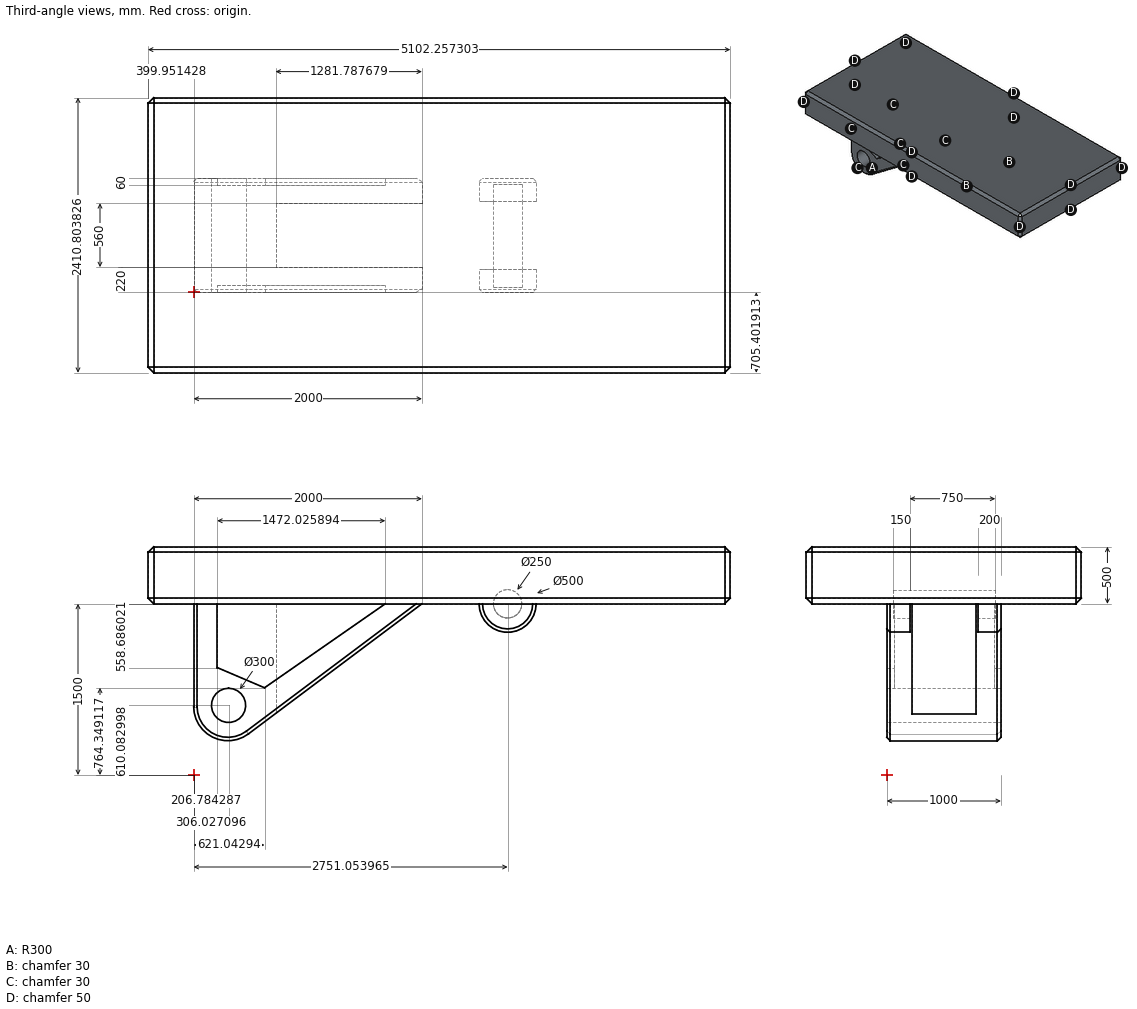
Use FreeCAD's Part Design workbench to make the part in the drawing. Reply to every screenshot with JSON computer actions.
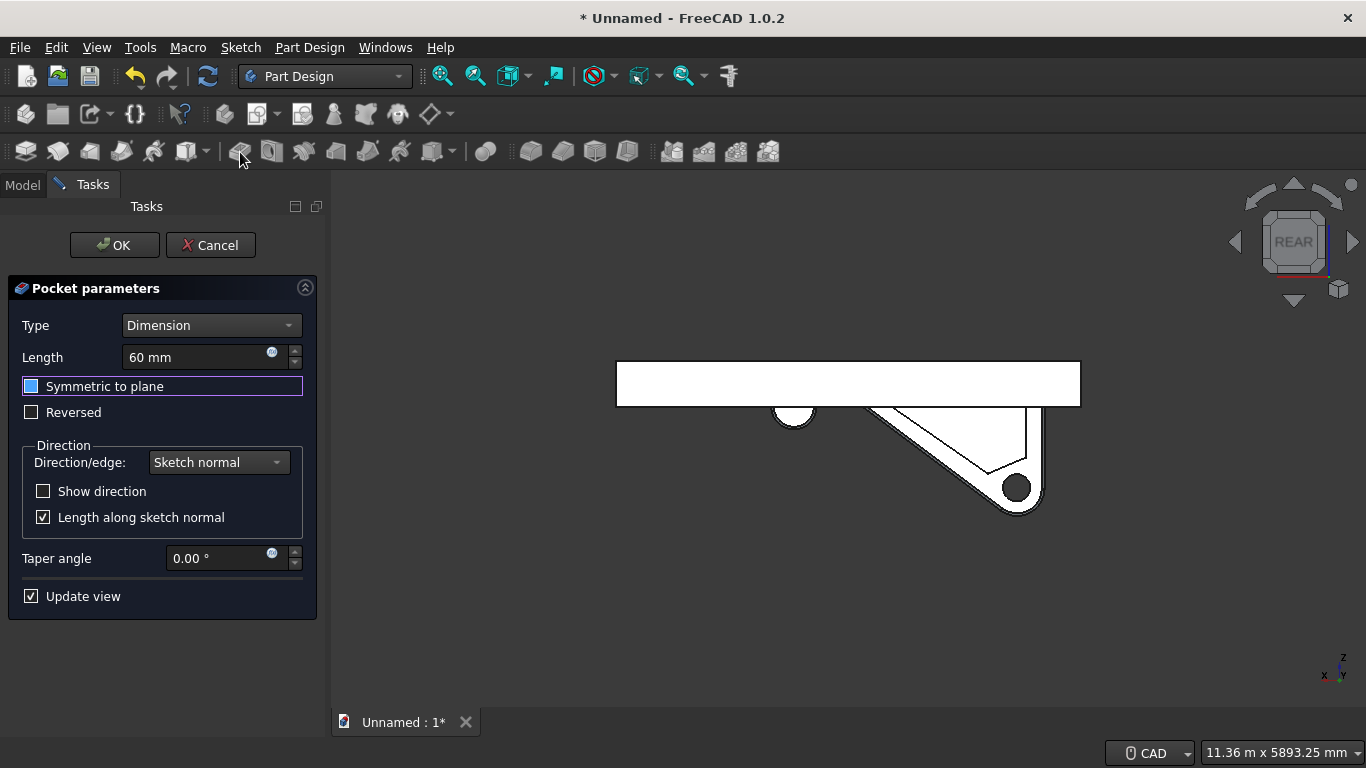
{"action": "left_click", "coordinate": [115, 245]}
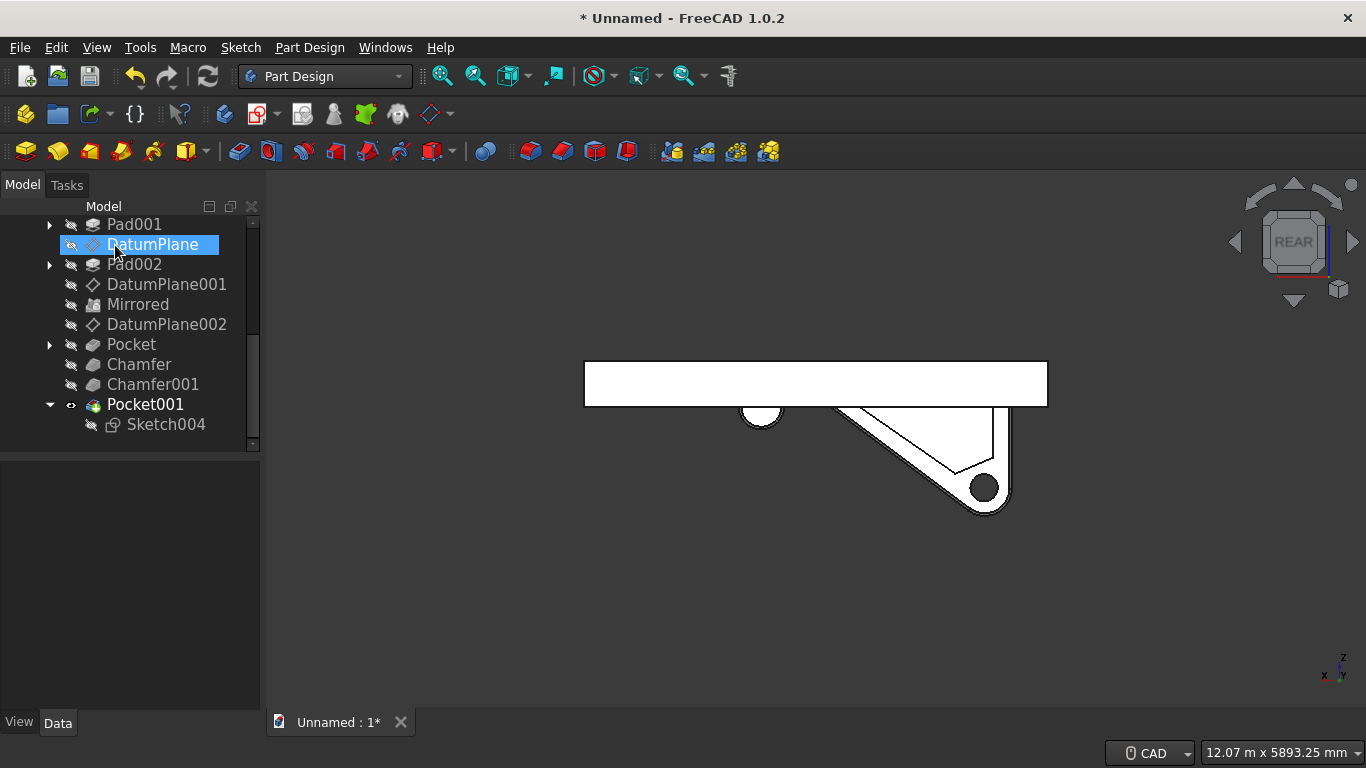
{"action": "left_click", "coordinate": [444, 76]}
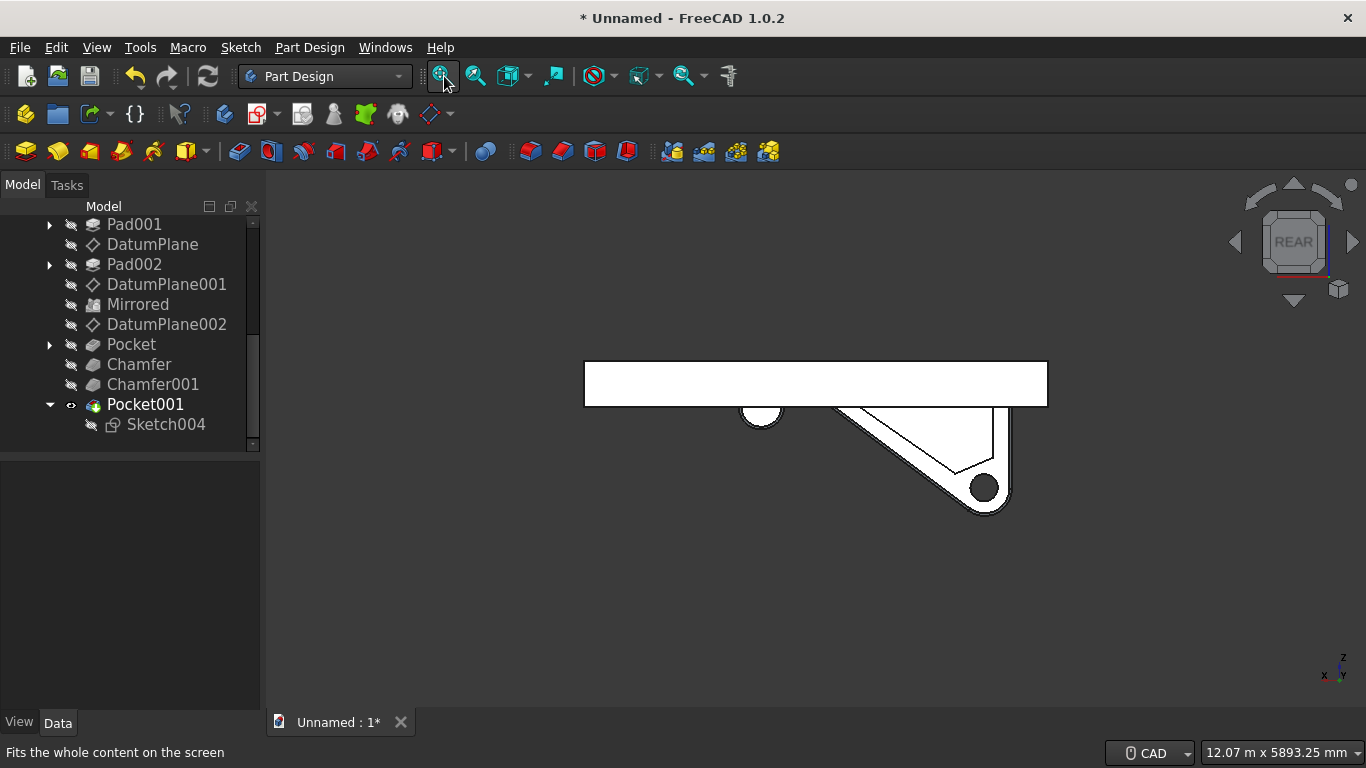
{"action": "scroll", "coordinate": [140, 320], "scroll_direction": "down", "scroll_amount": 3}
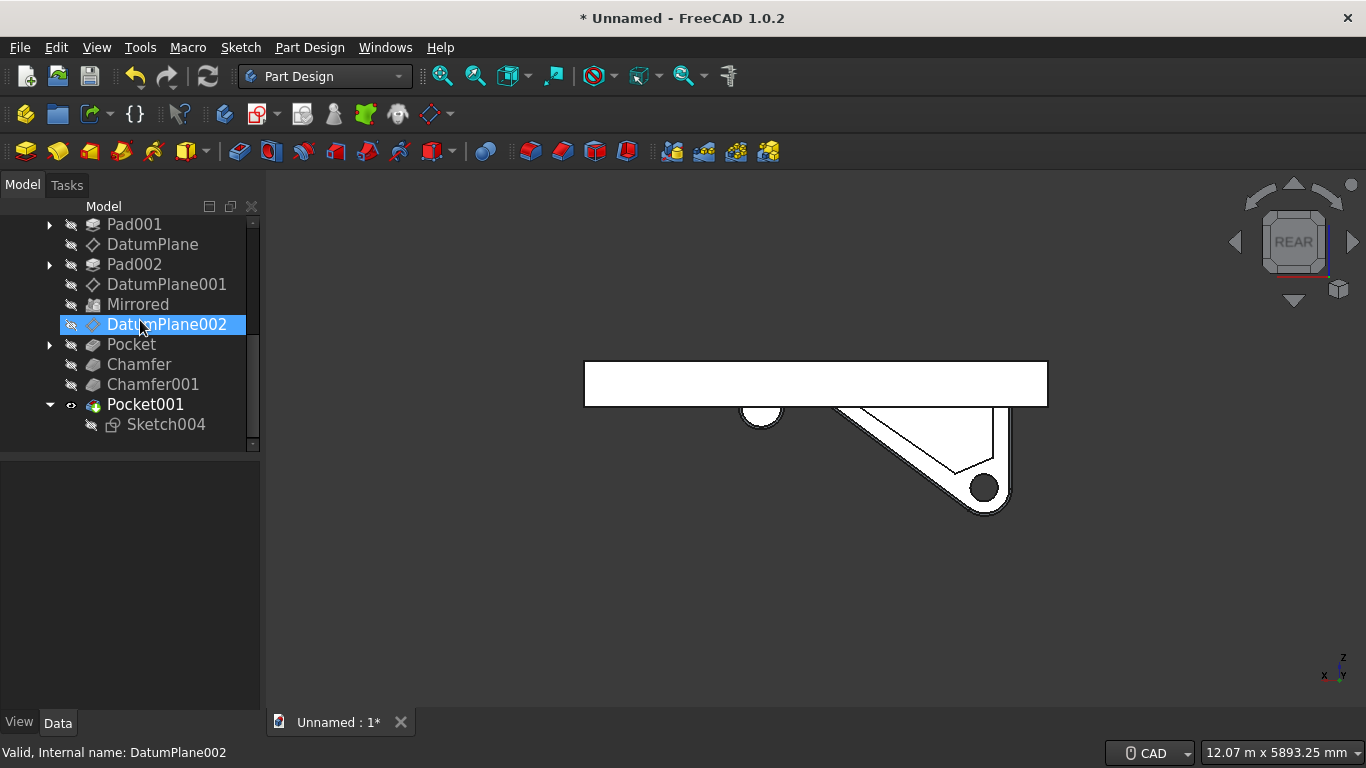
{"action": "scroll", "coordinate": [140, 320], "scroll_direction": "up", "scroll_amount": 15}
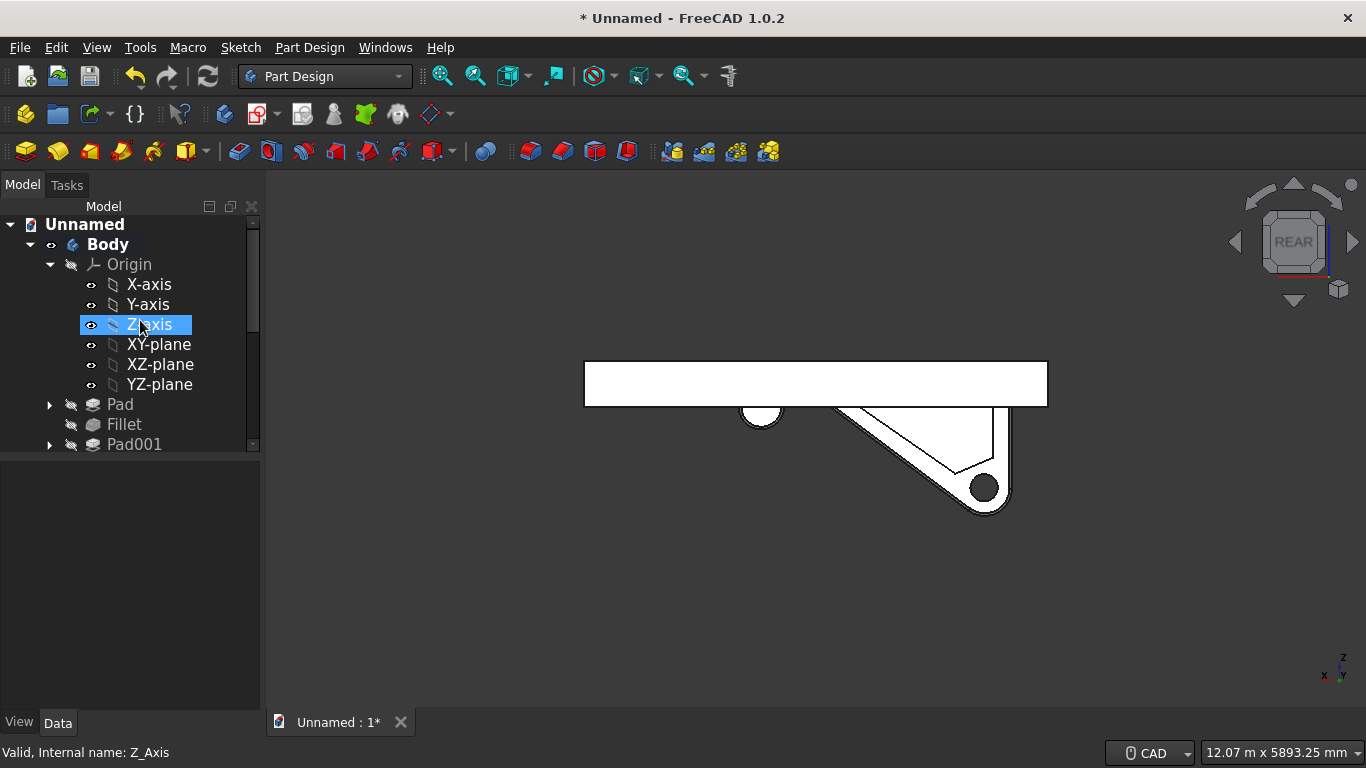
{"action": "left_click", "coordinate": [136, 365]}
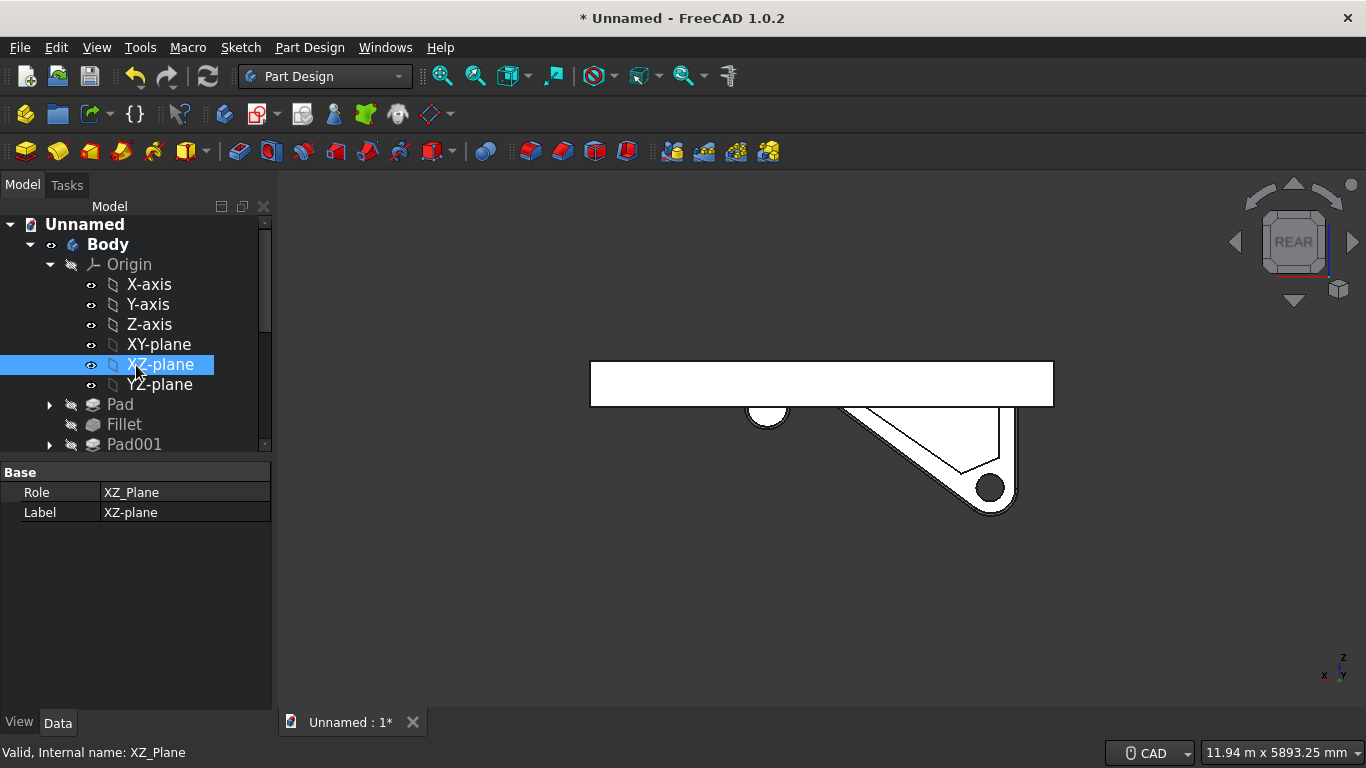
{"action": "left_click", "coordinate": [430, 114]}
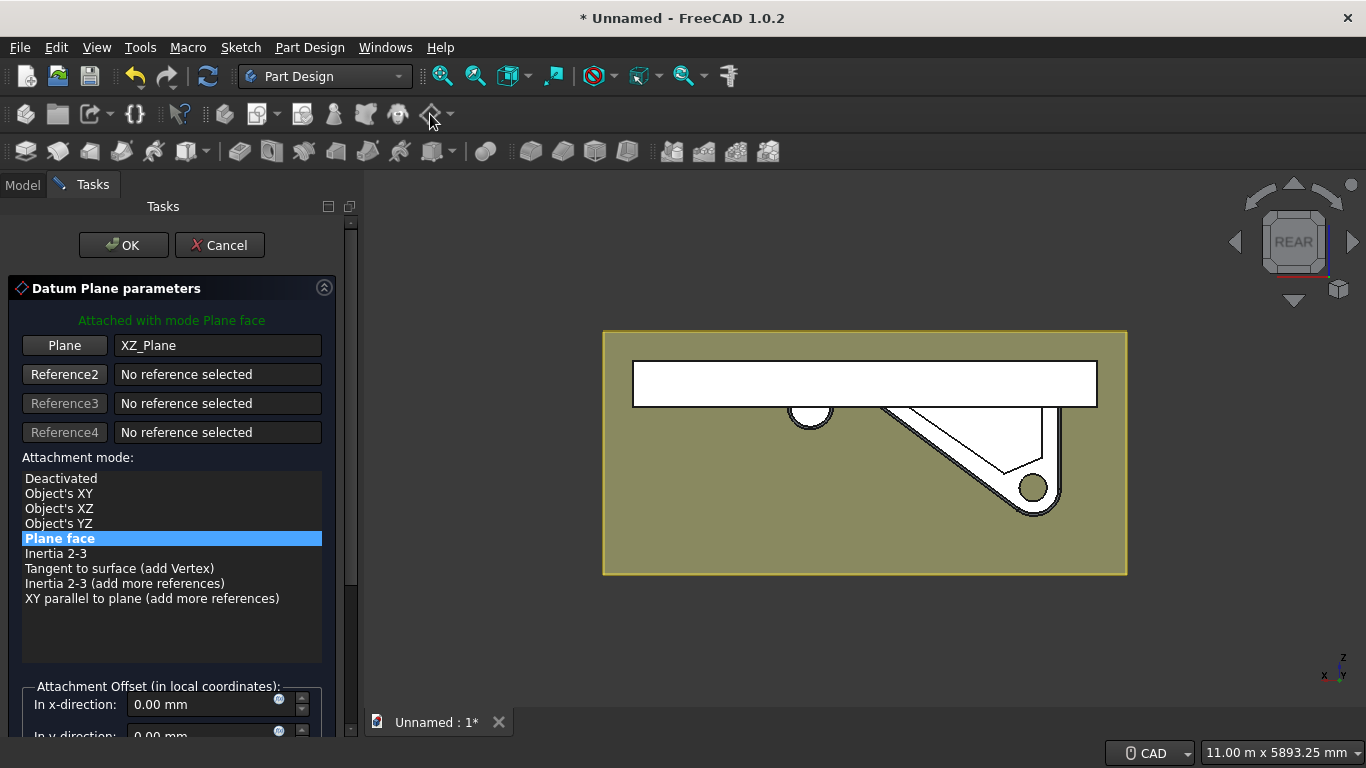
{"action": "scroll", "coordinate": [351, 476], "scroll_direction": "down", "scroll_amount": 2}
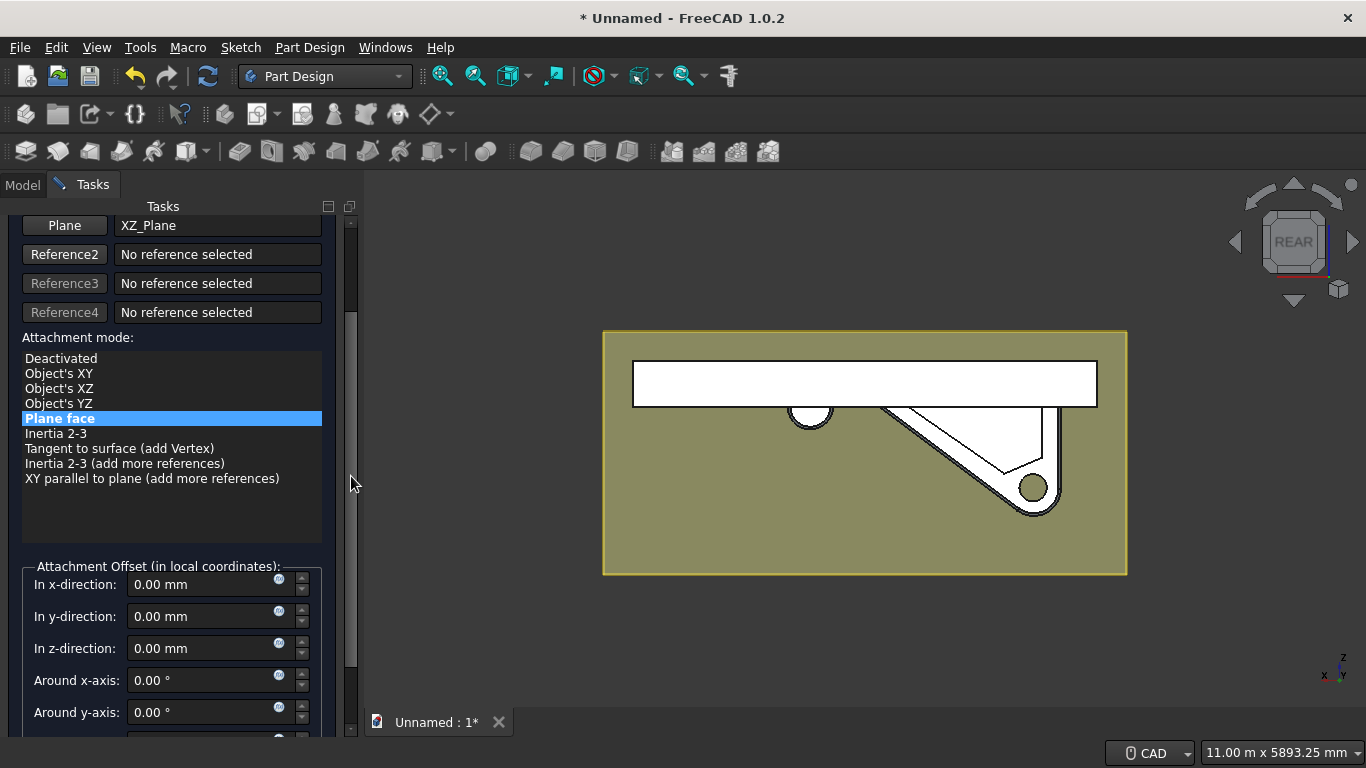
{"action": "triple_click", "coordinate": [210, 648]}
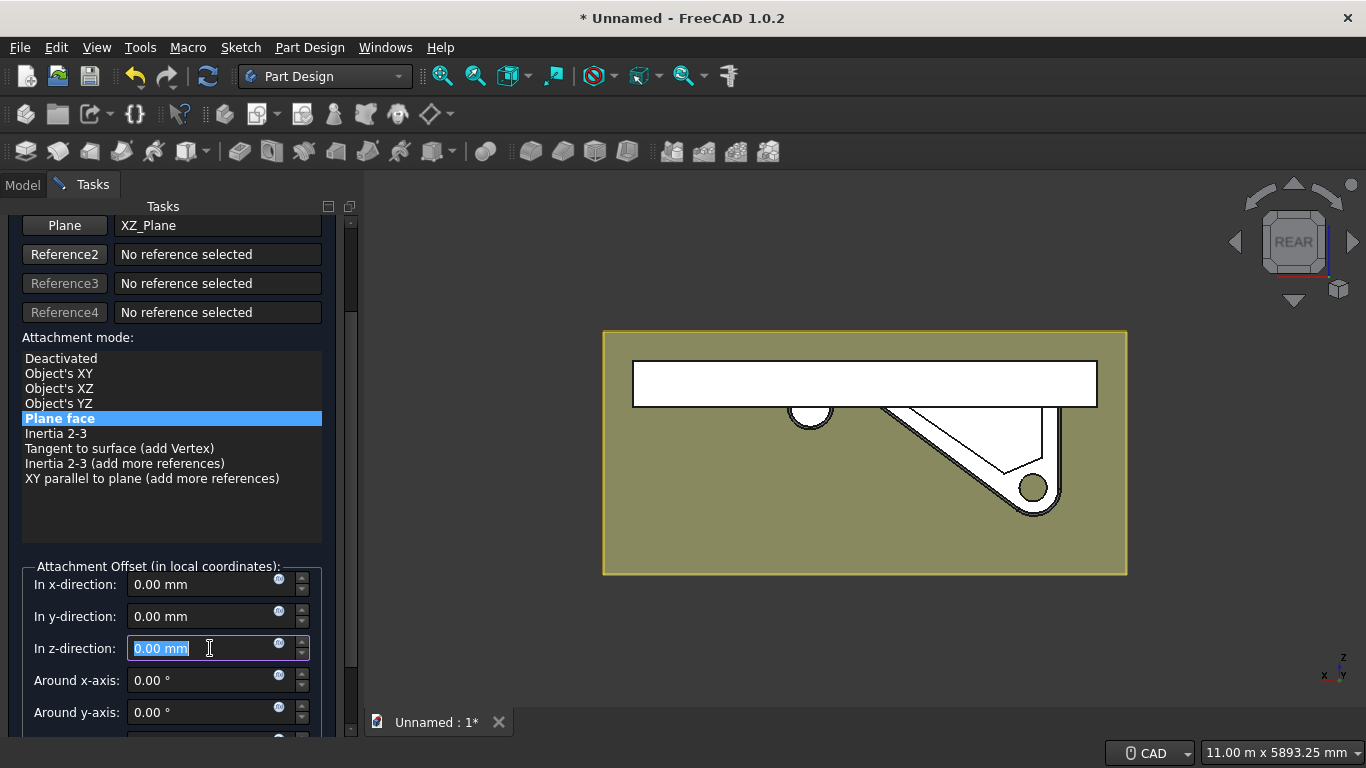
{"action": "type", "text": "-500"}
{"action": "key", "text": "Tab"}